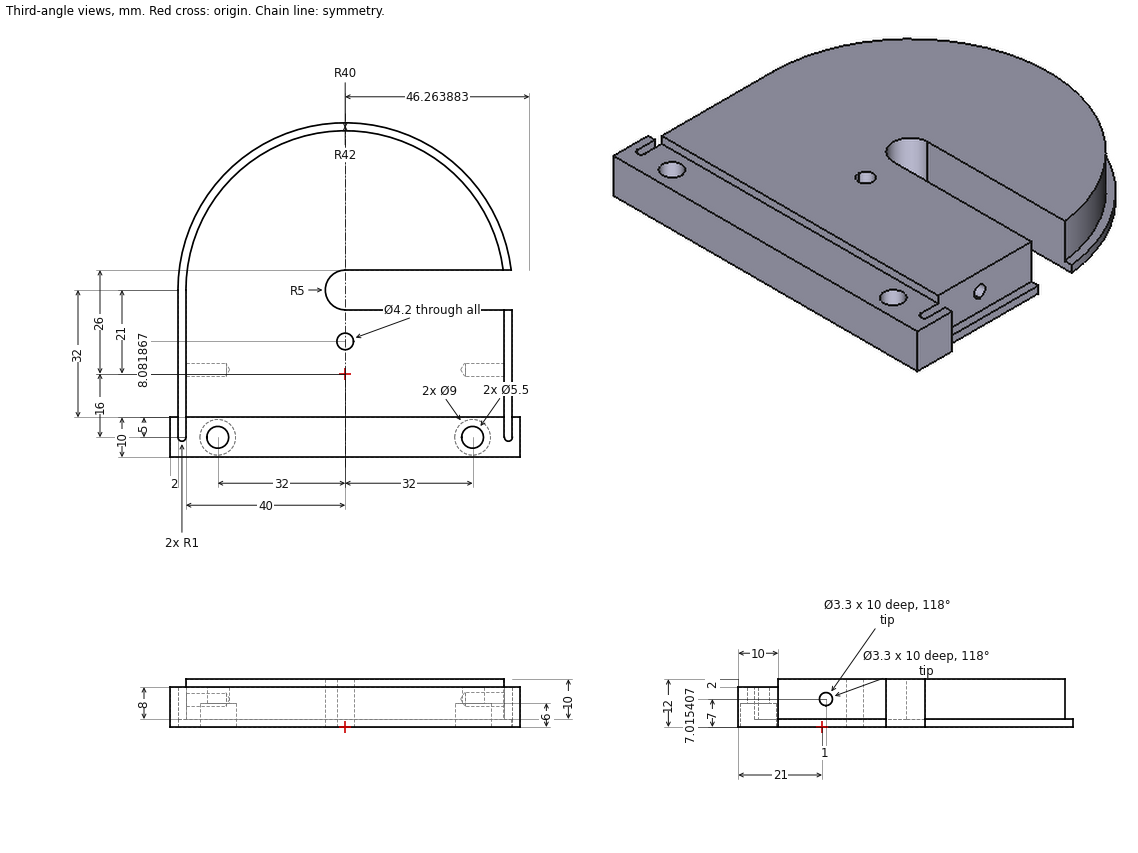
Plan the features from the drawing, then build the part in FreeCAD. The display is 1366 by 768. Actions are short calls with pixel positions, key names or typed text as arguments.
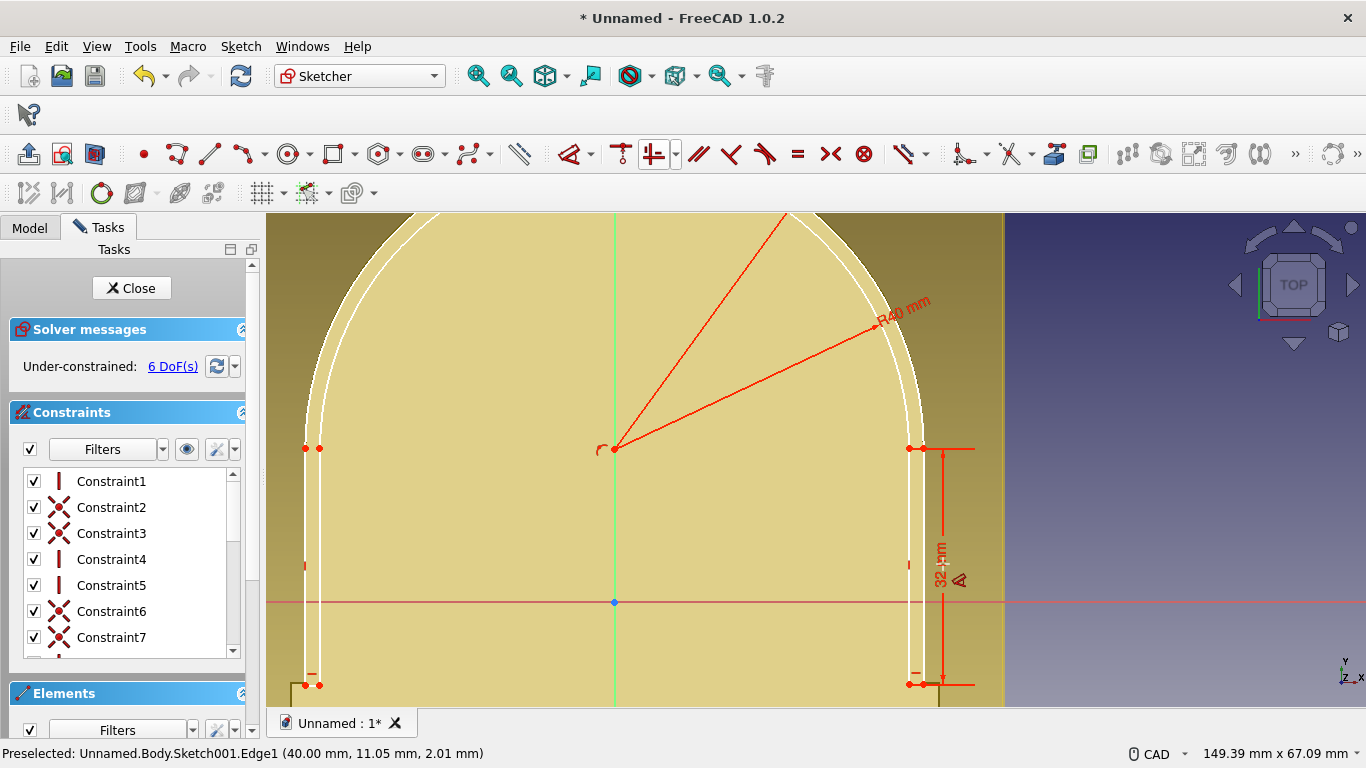
click(924, 614)
click(958, 511)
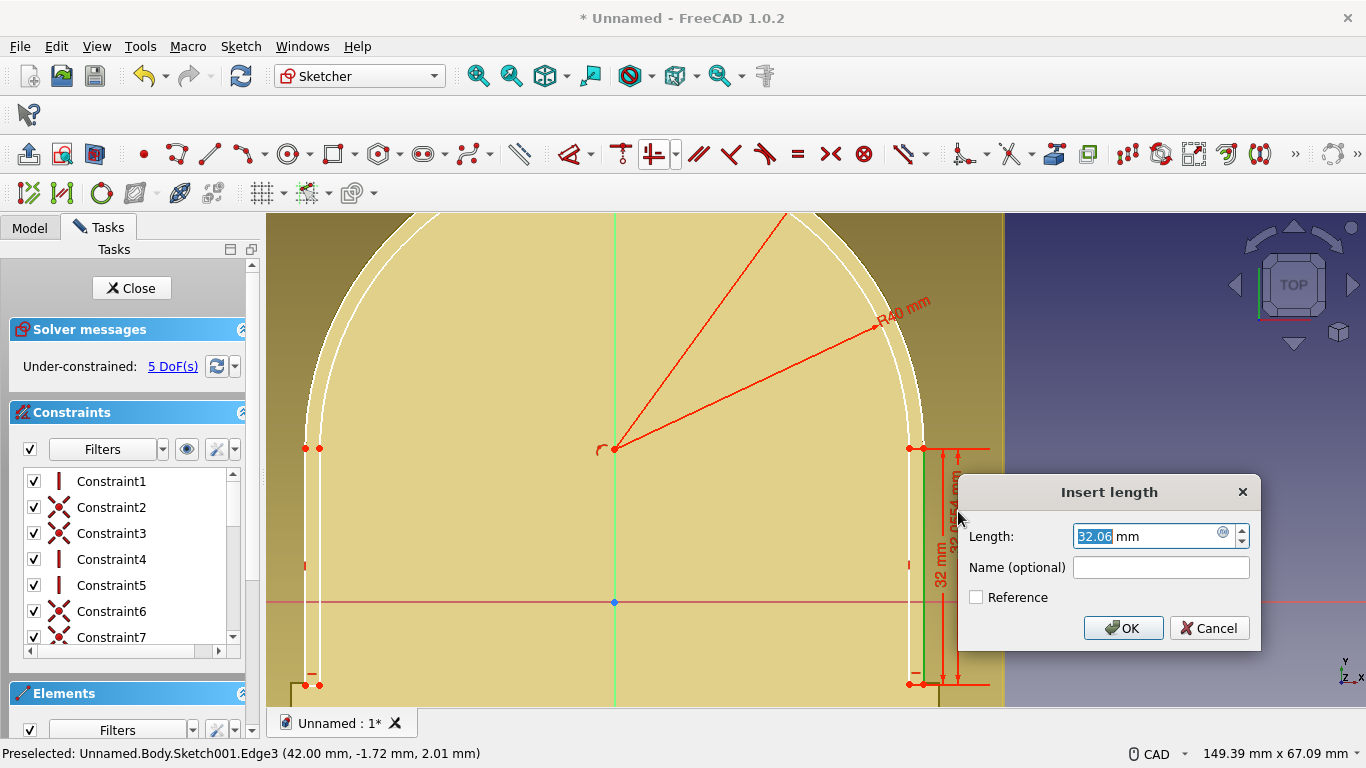
text(32)
key(Return)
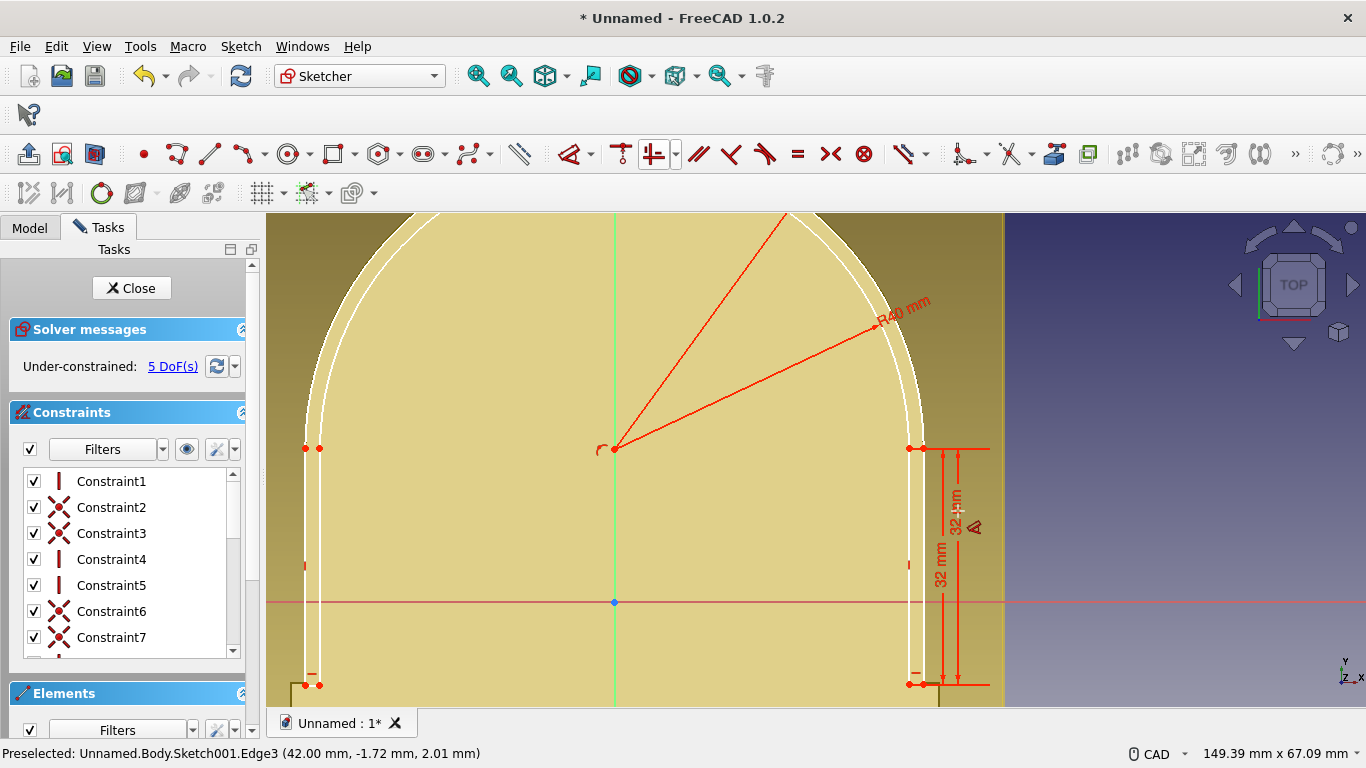
click(305, 520)
click(339, 564)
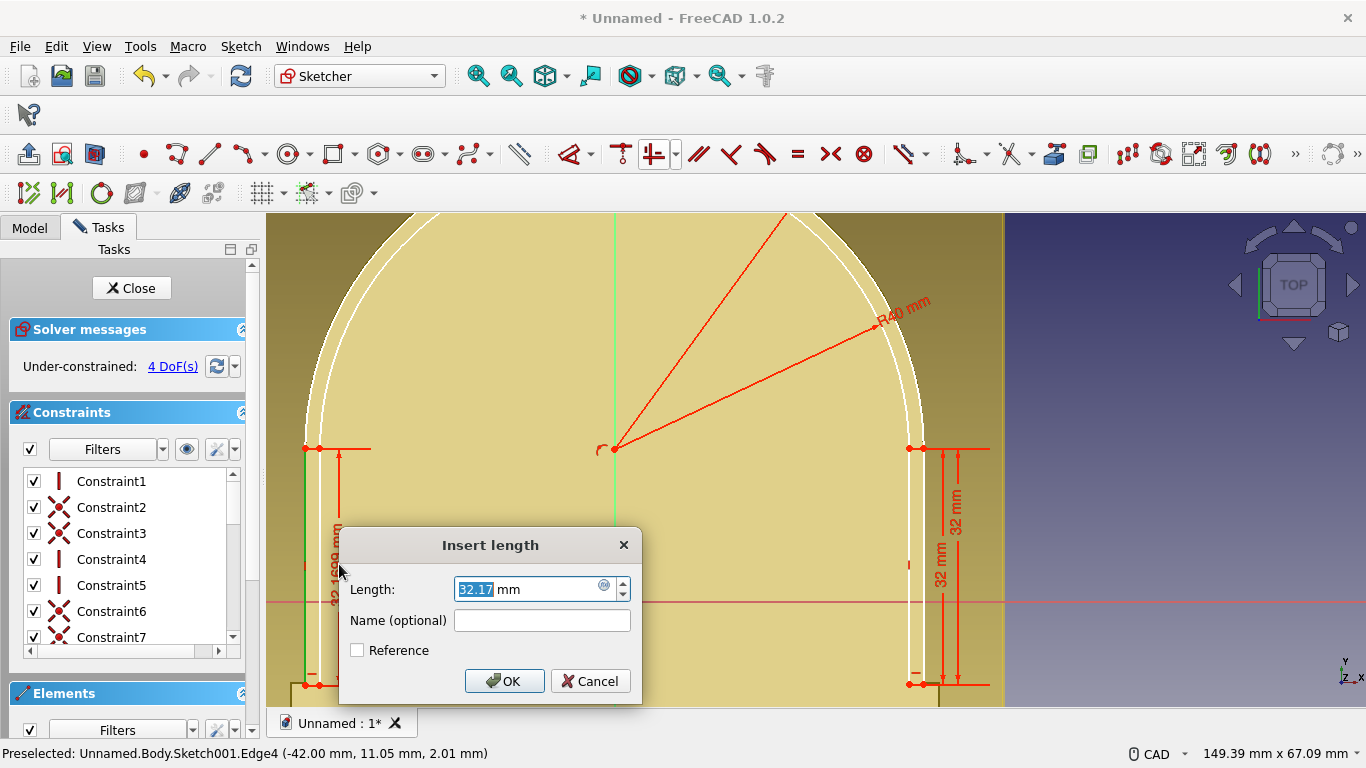
text(32)
key(Return)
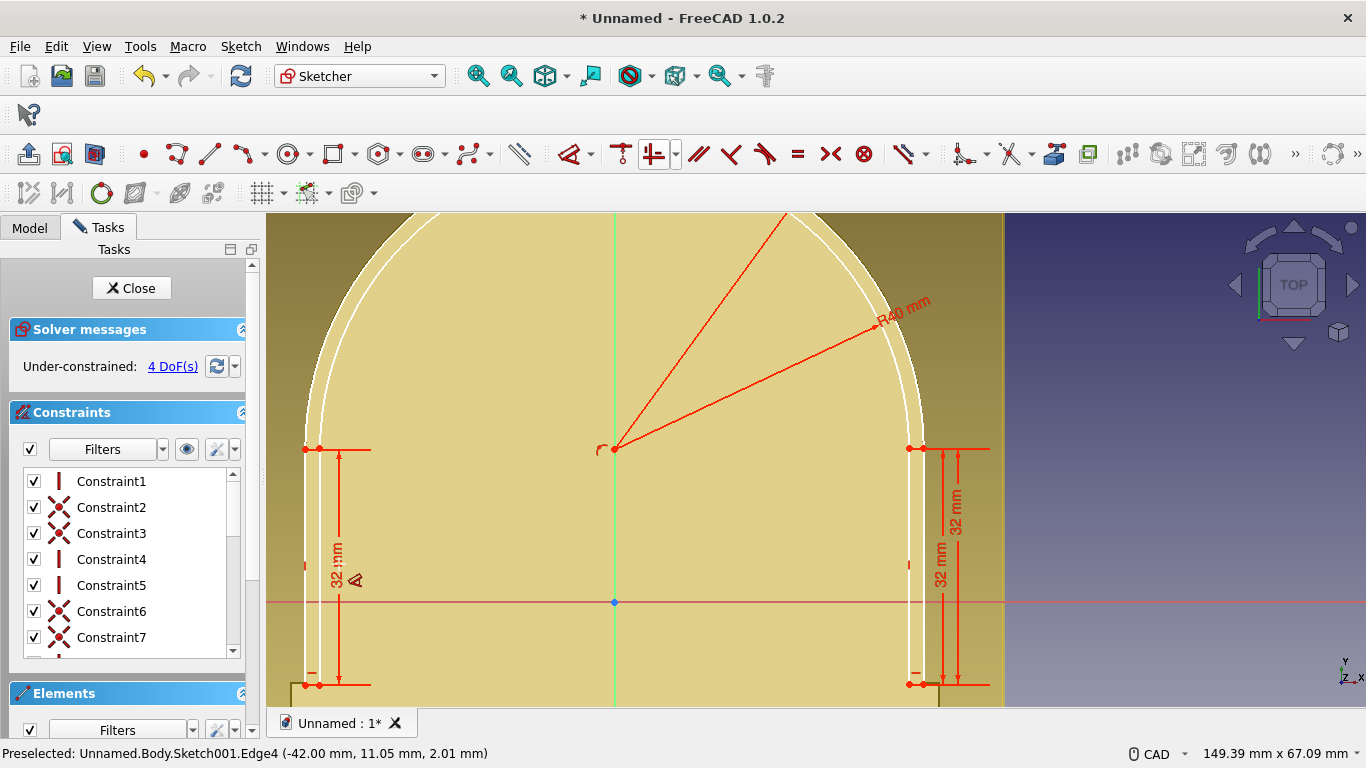
click(320, 614)
click(354, 511)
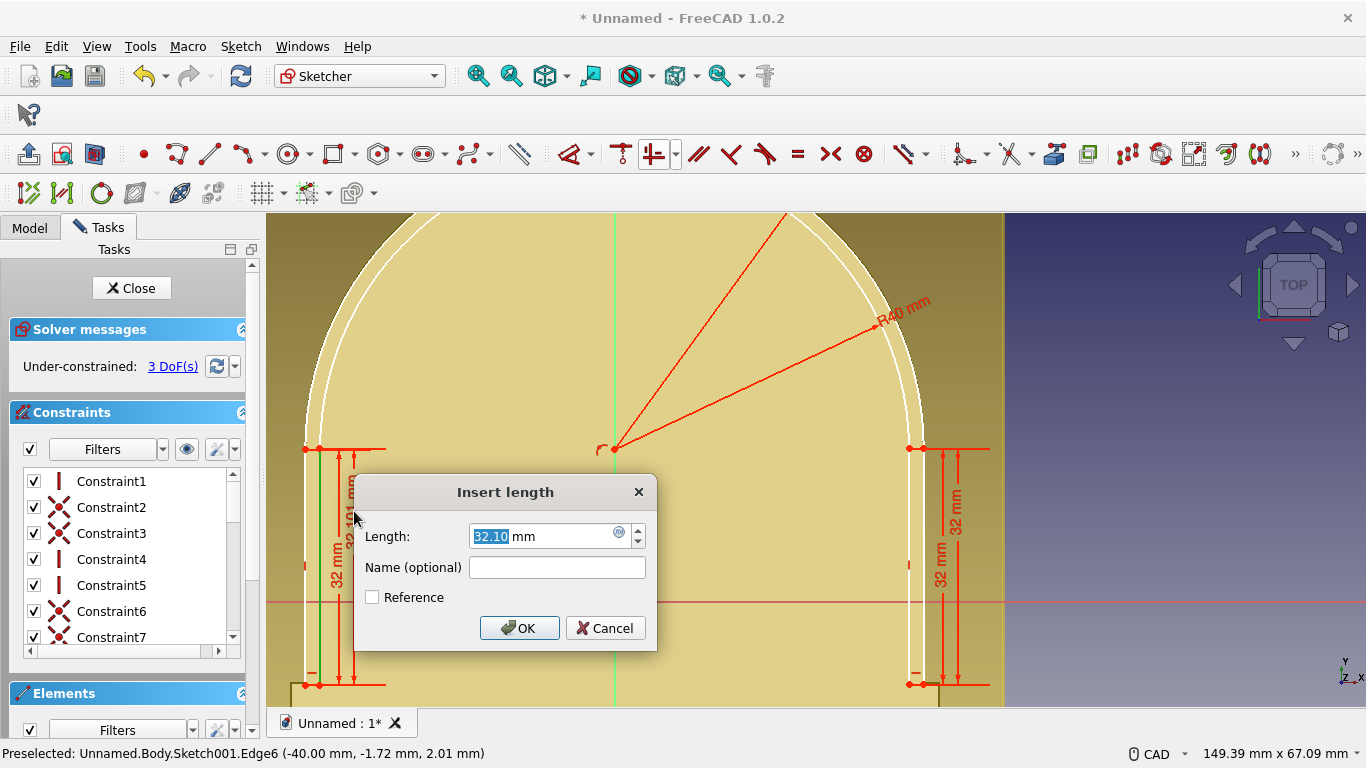
text(32)
key(Return)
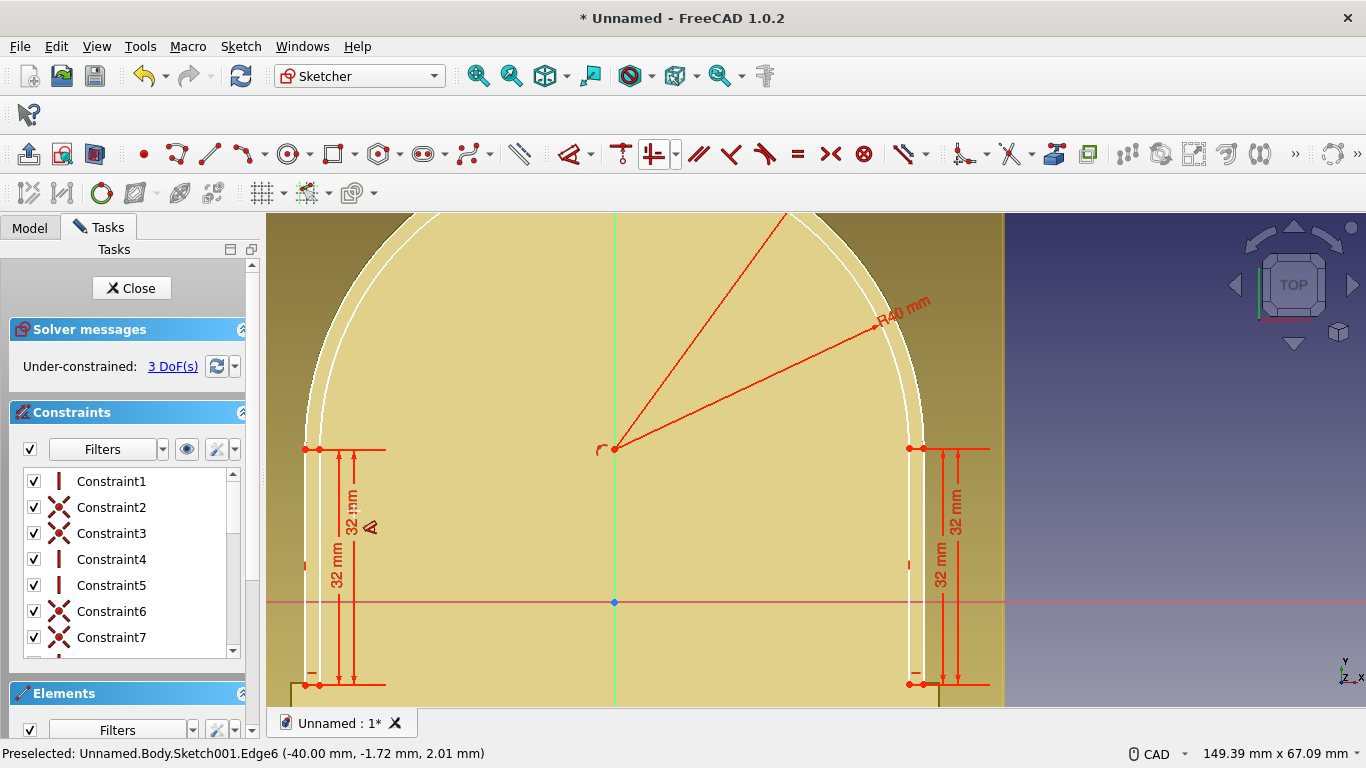
click(909, 449)
click(943, 490)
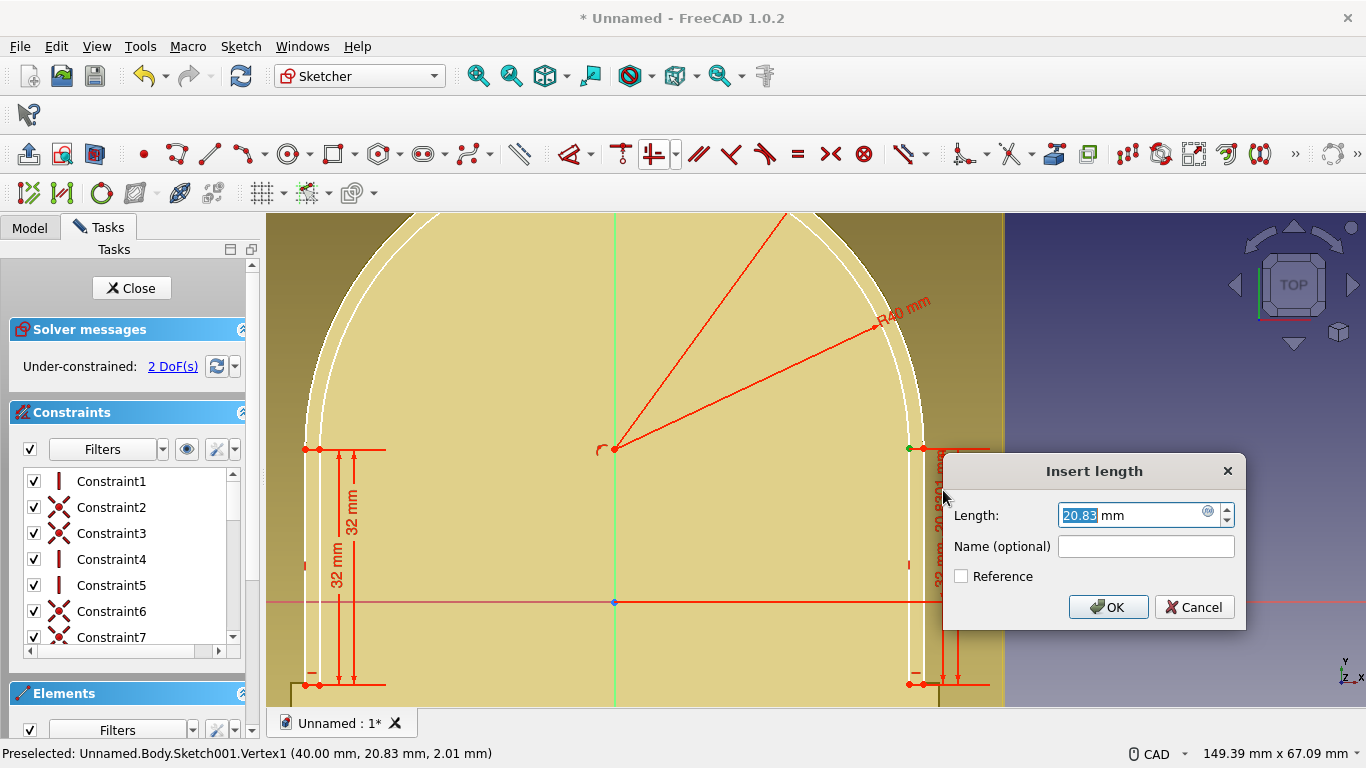
text(21)
key(Return)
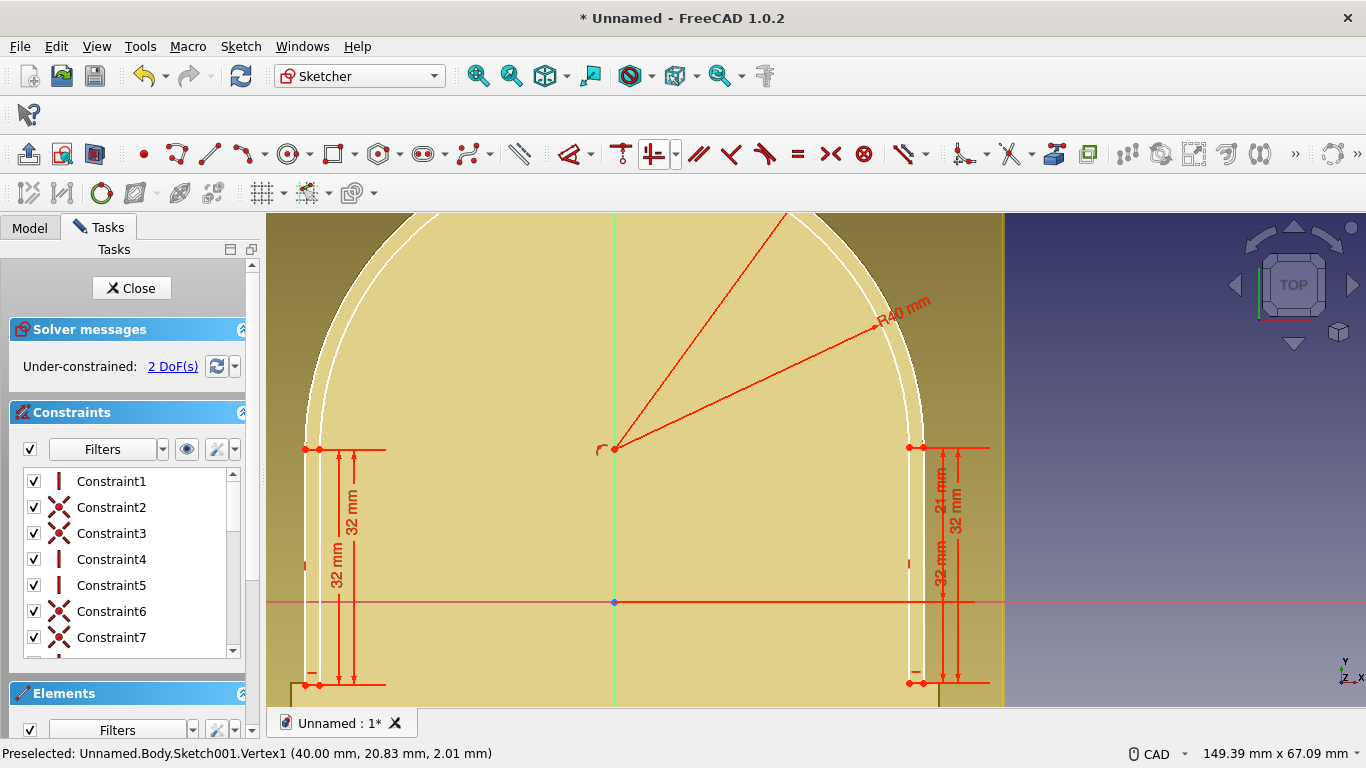
click(305, 450)
click(649, 526)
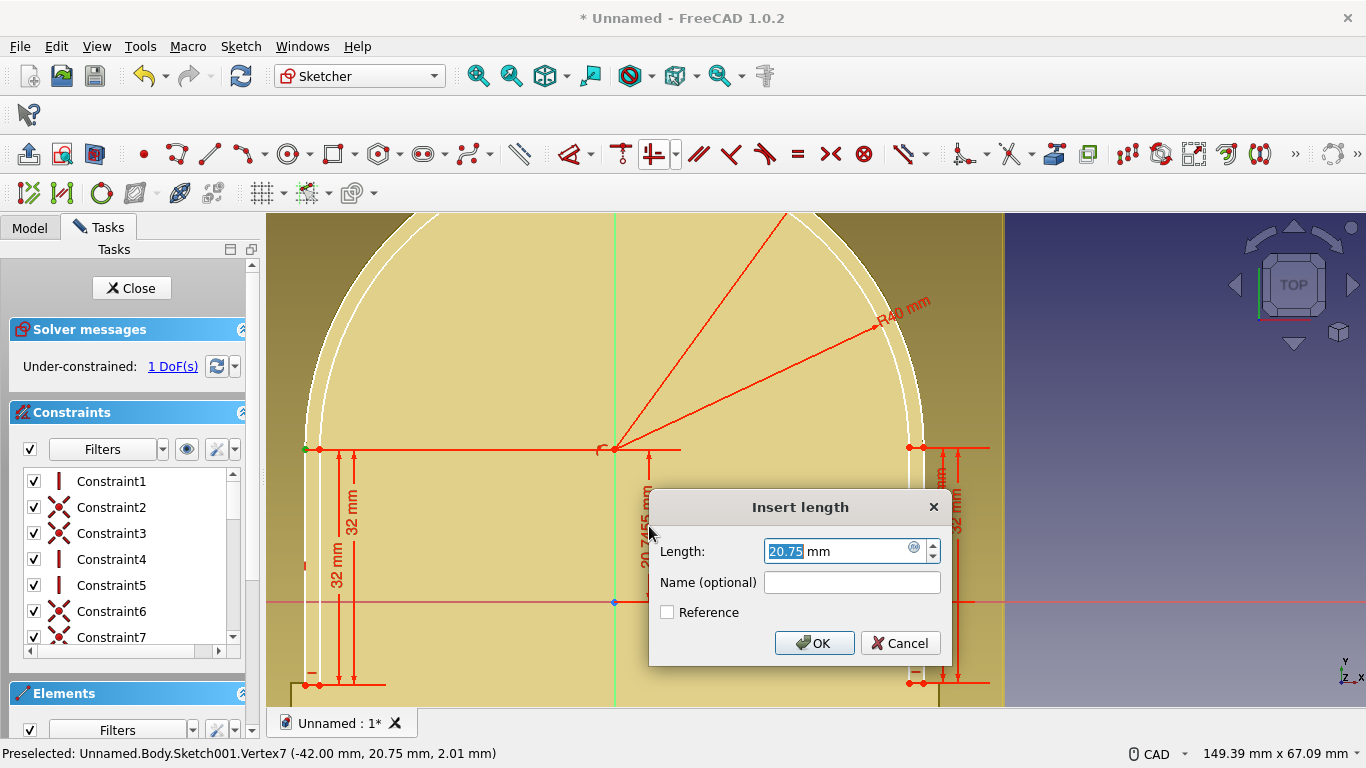
text(21)
key(Return)